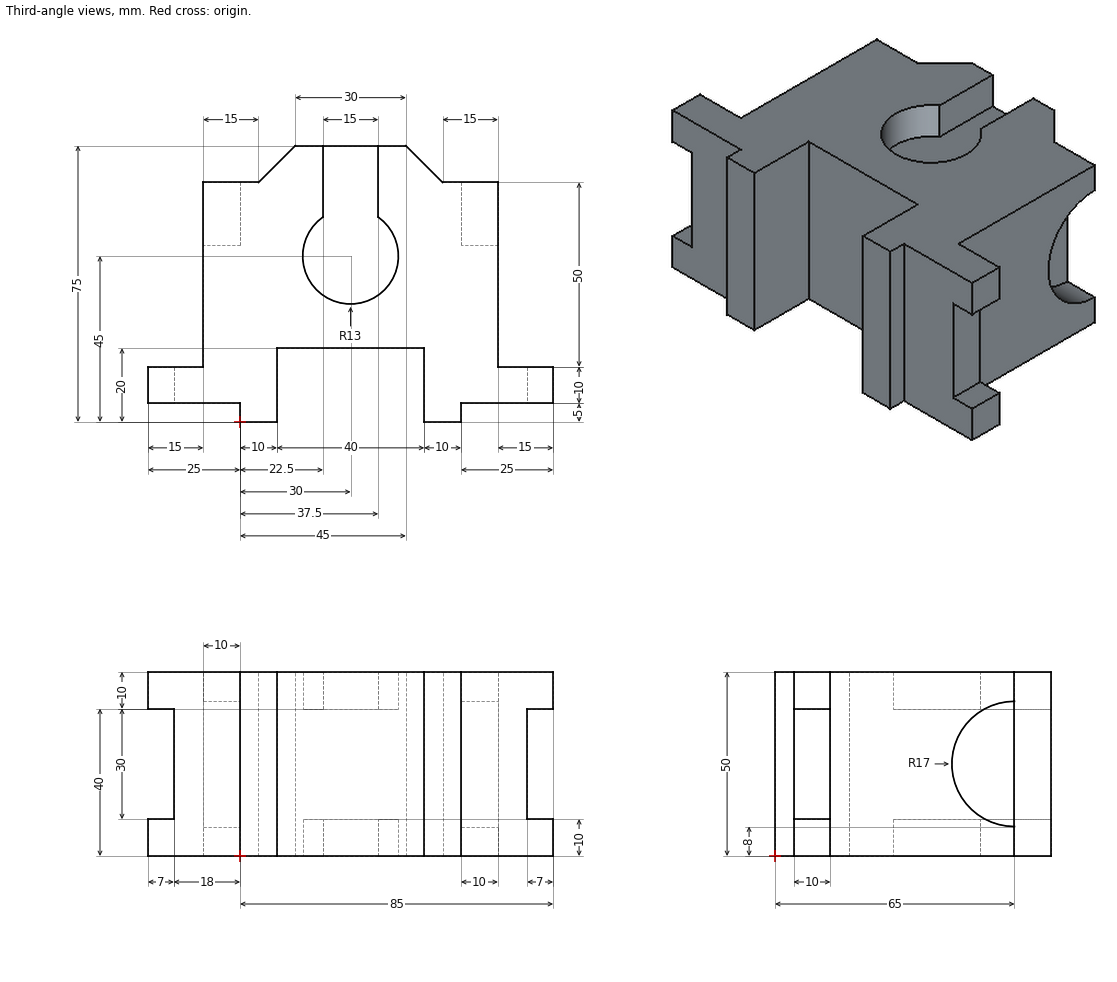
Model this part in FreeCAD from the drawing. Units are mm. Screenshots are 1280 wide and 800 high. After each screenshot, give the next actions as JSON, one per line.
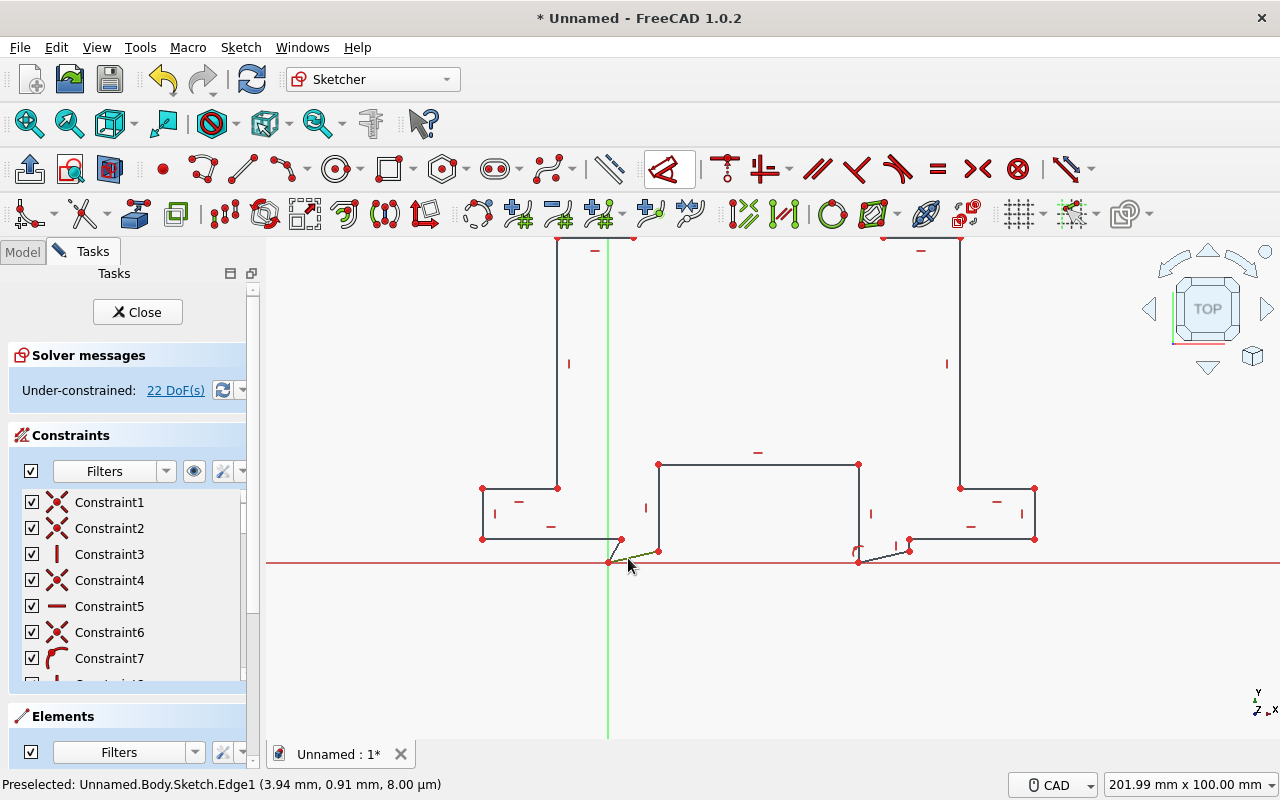
{"action": "left_click", "coordinate": [792, 170]}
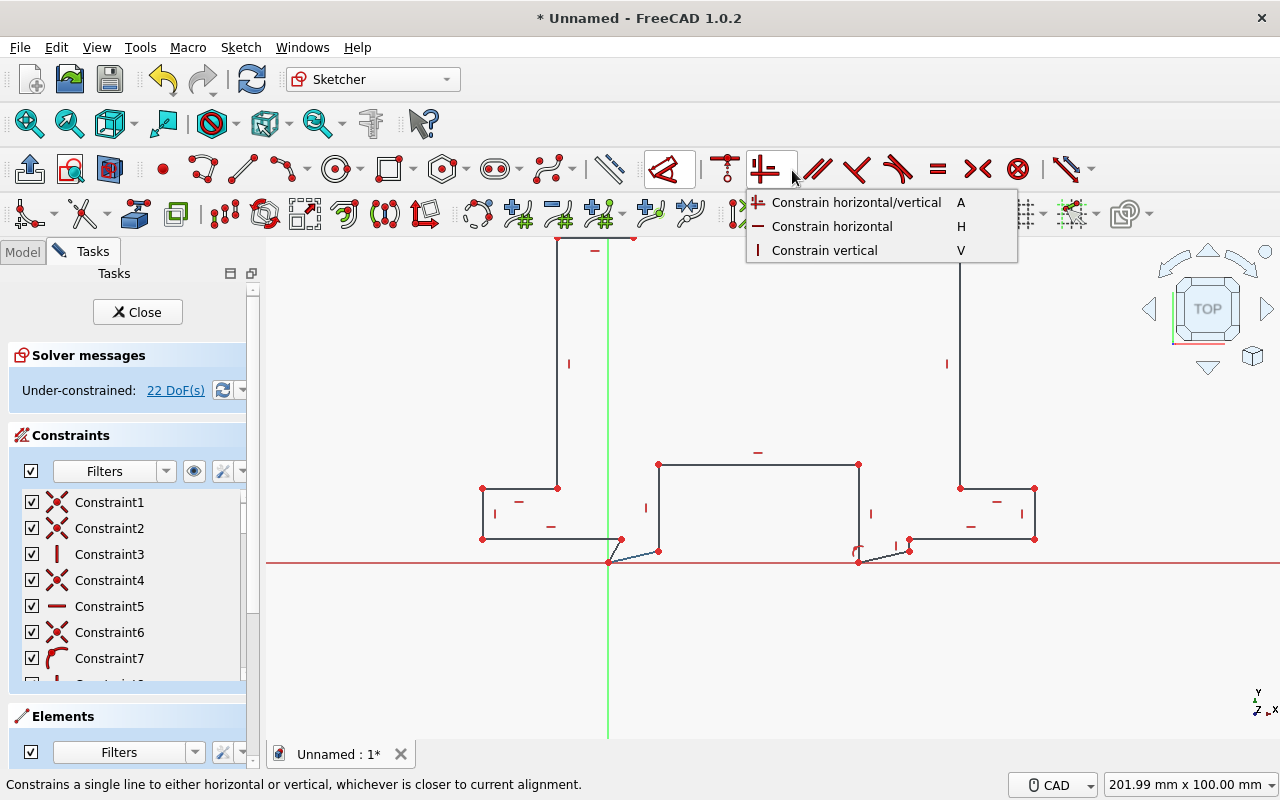
{"action": "left_click", "coordinate": [882, 226]}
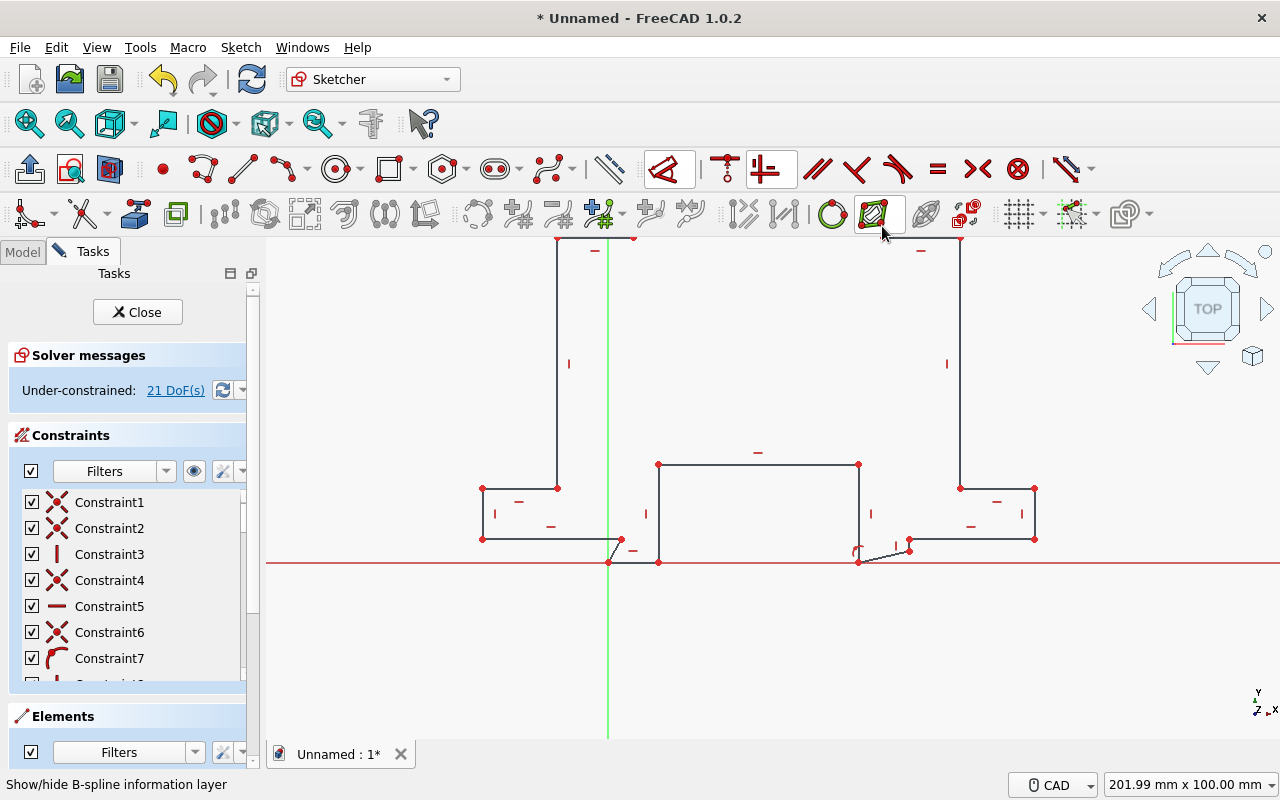
{"action": "left_click", "coordinate": [874, 559]}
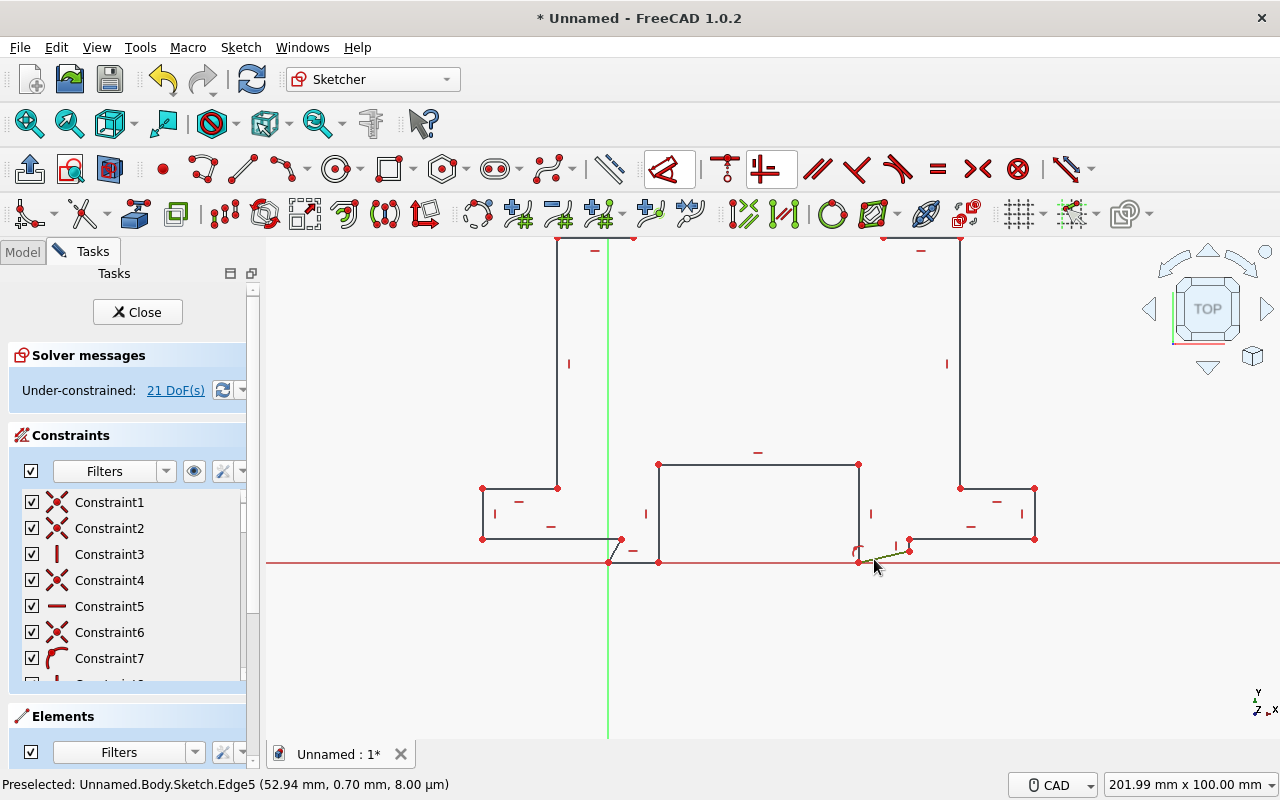
{"action": "key", "text": "h"}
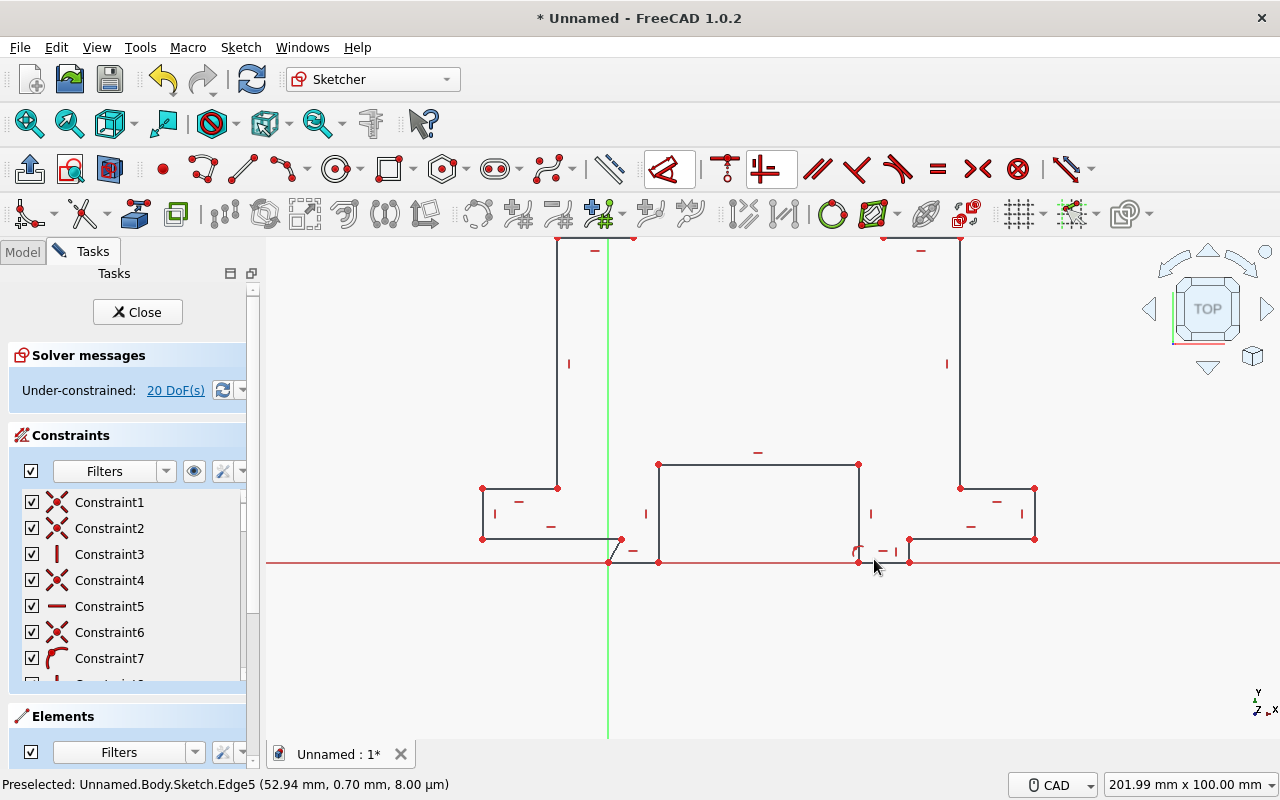
{"action": "scroll", "coordinate": [616, 549], "scroll_direction": "up", "scroll_amount": 3}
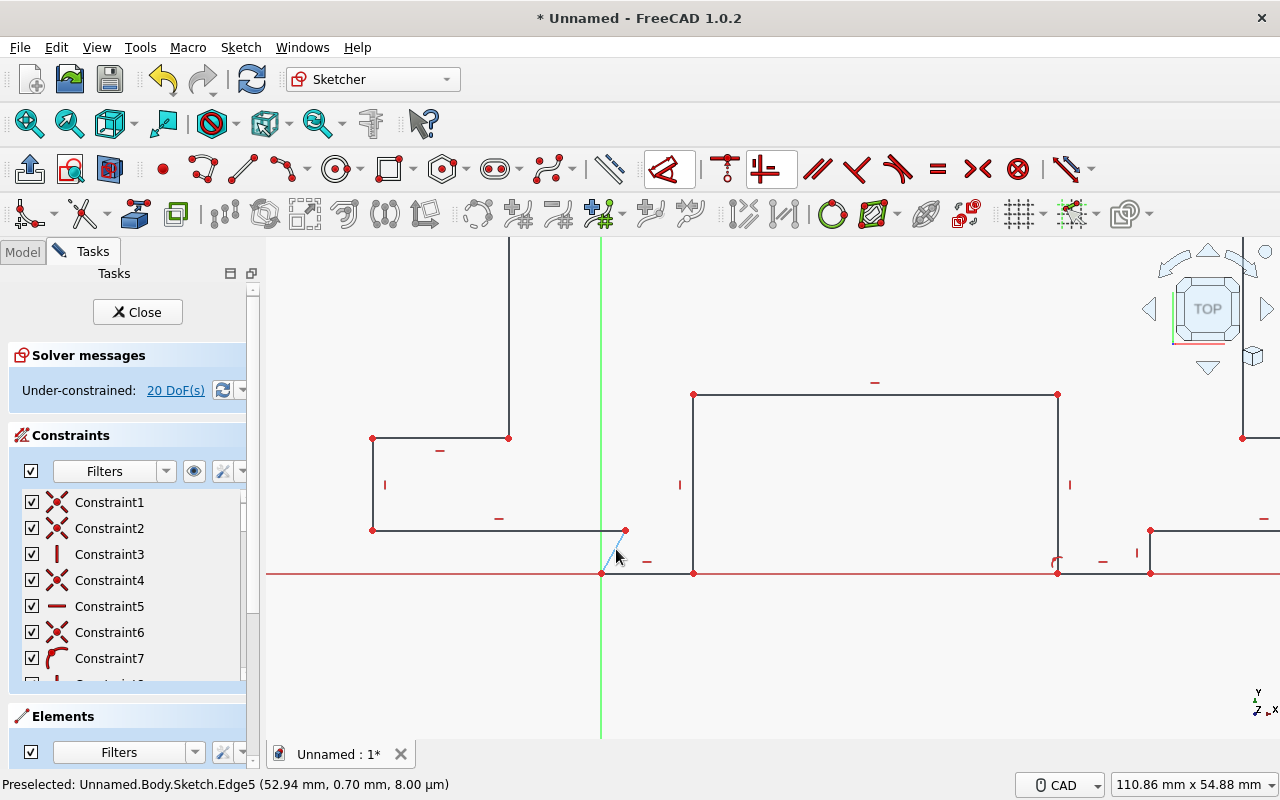
{"action": "left_click", "coordinate": [616, 548]}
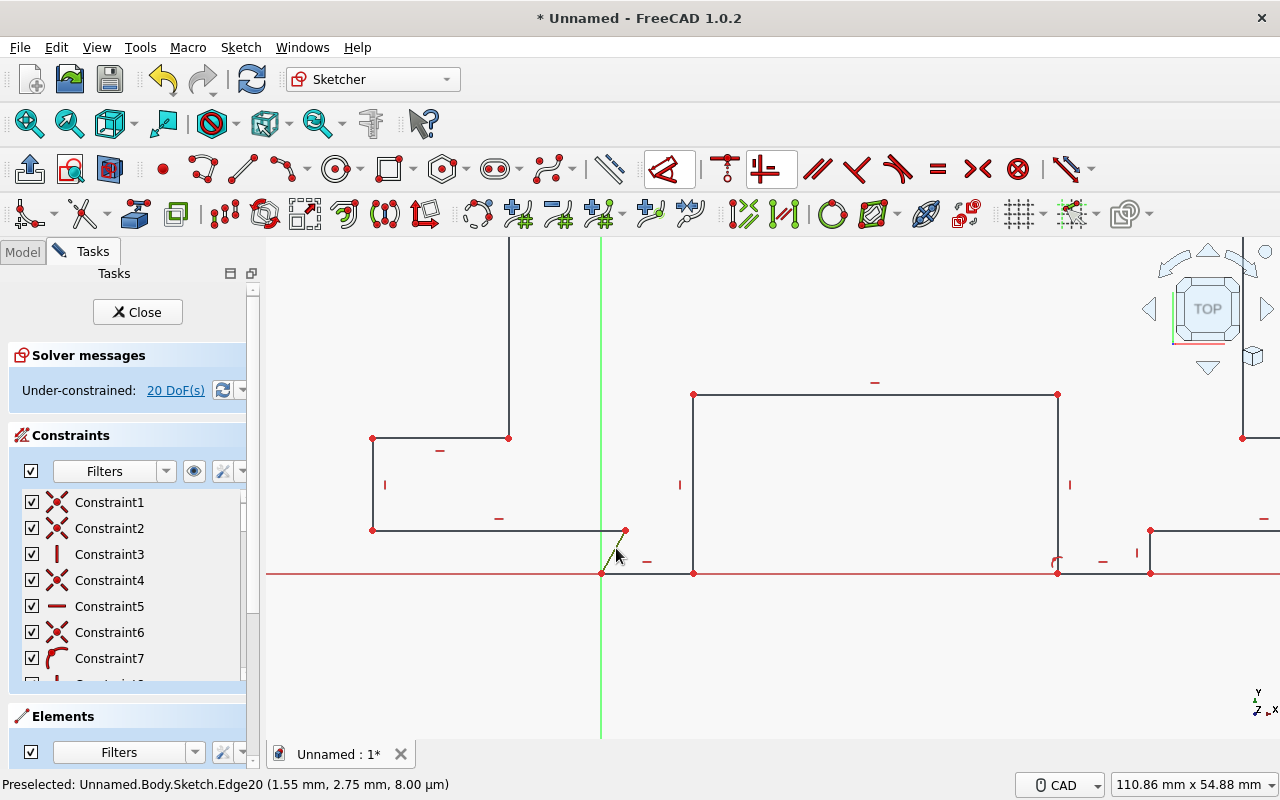
{"action": "left_click", "coordinate": [792, 170]}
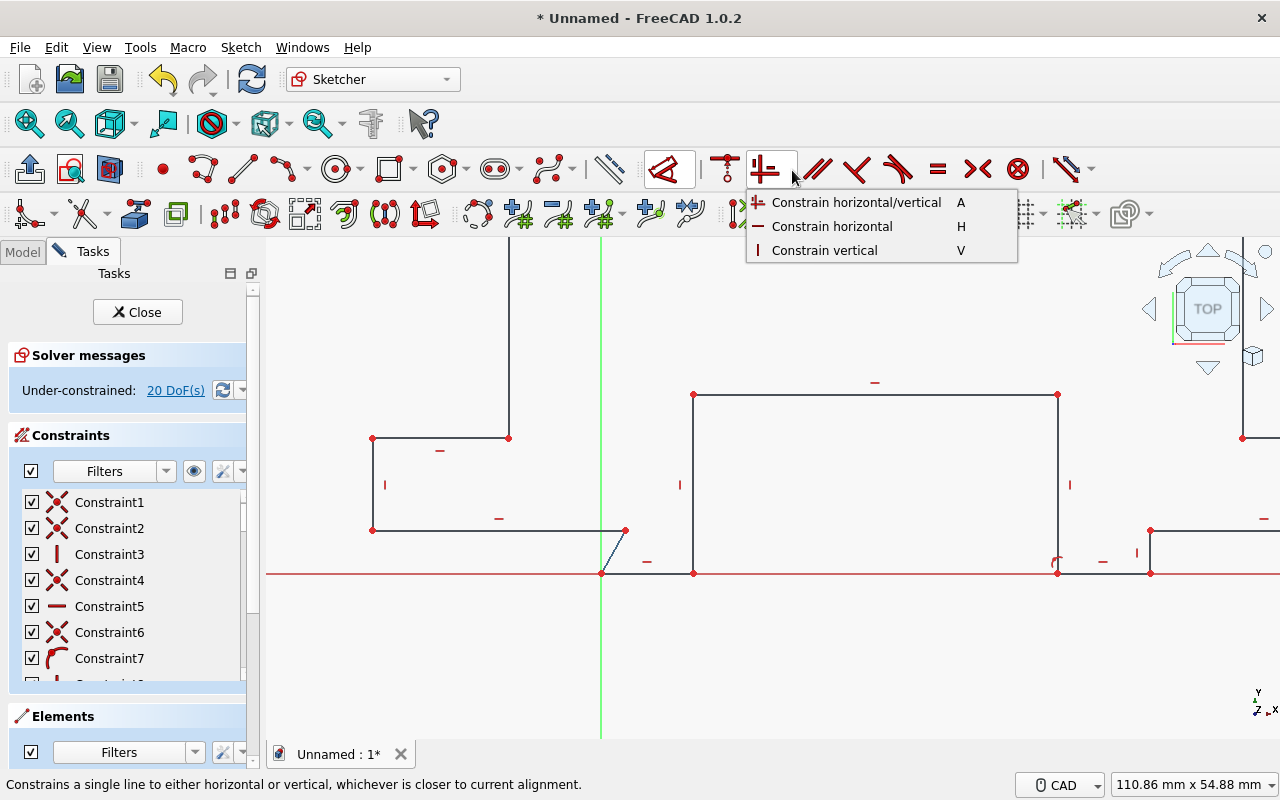
{"action": "left_click", "coordinate": [882, 250]}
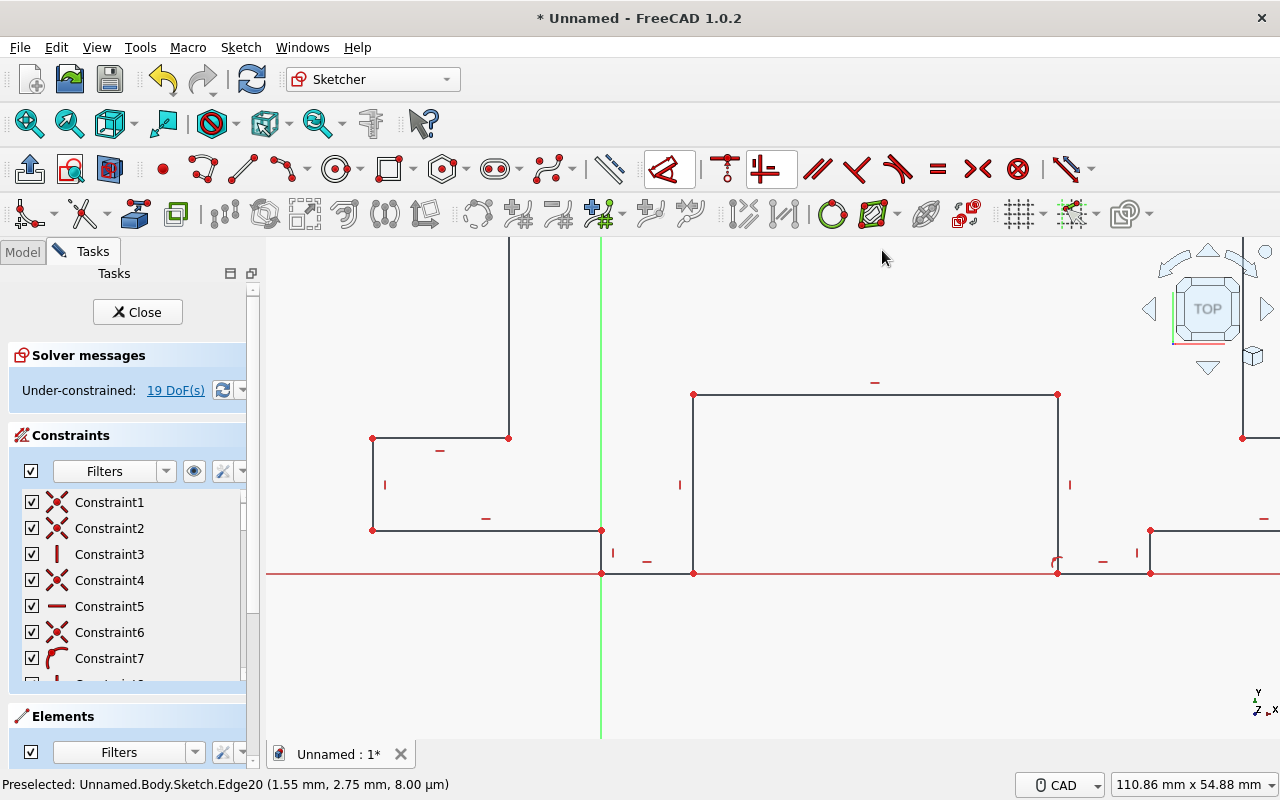
{"action": "left_click", "coordinate": [664, 170]}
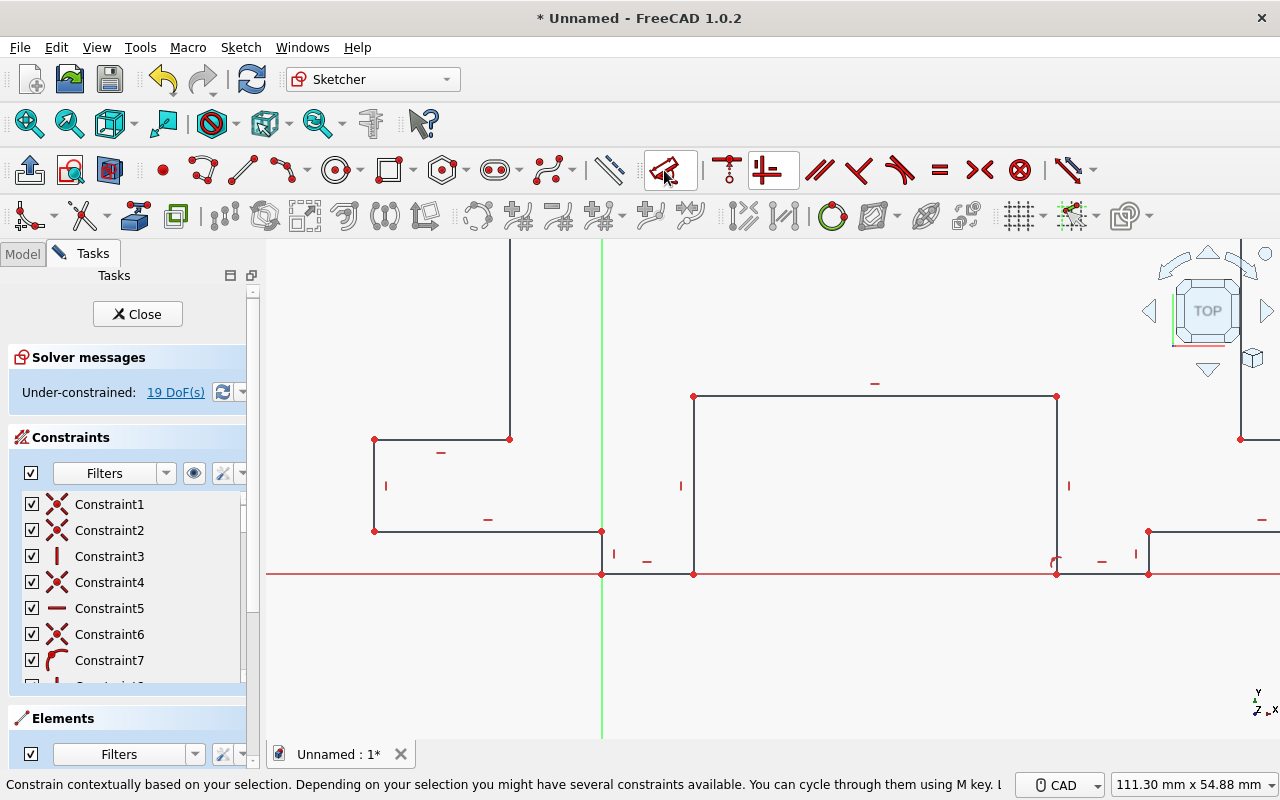
{"action": "scroll", "coordinate": [565, 698], "scroll_direction": "down", "scroll_amount": 4}